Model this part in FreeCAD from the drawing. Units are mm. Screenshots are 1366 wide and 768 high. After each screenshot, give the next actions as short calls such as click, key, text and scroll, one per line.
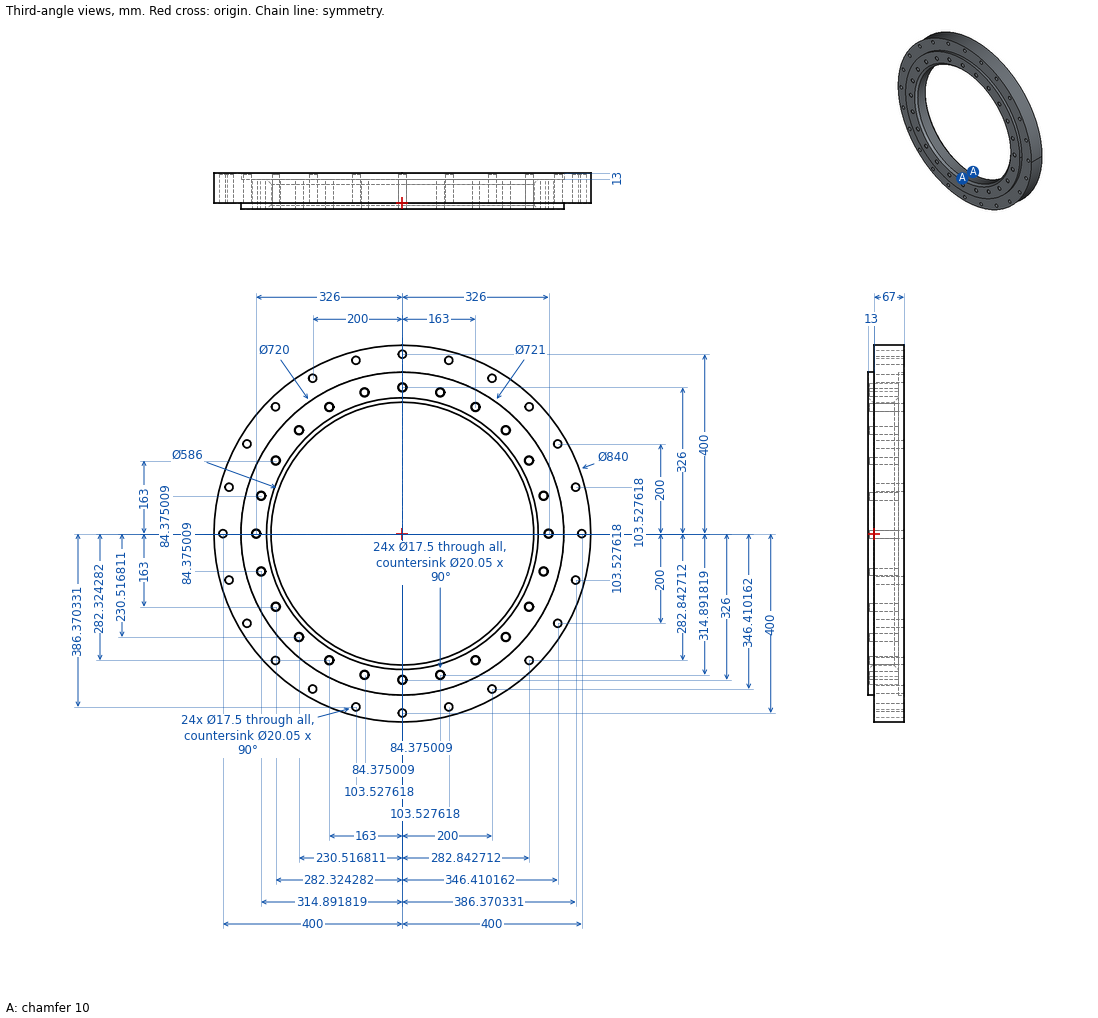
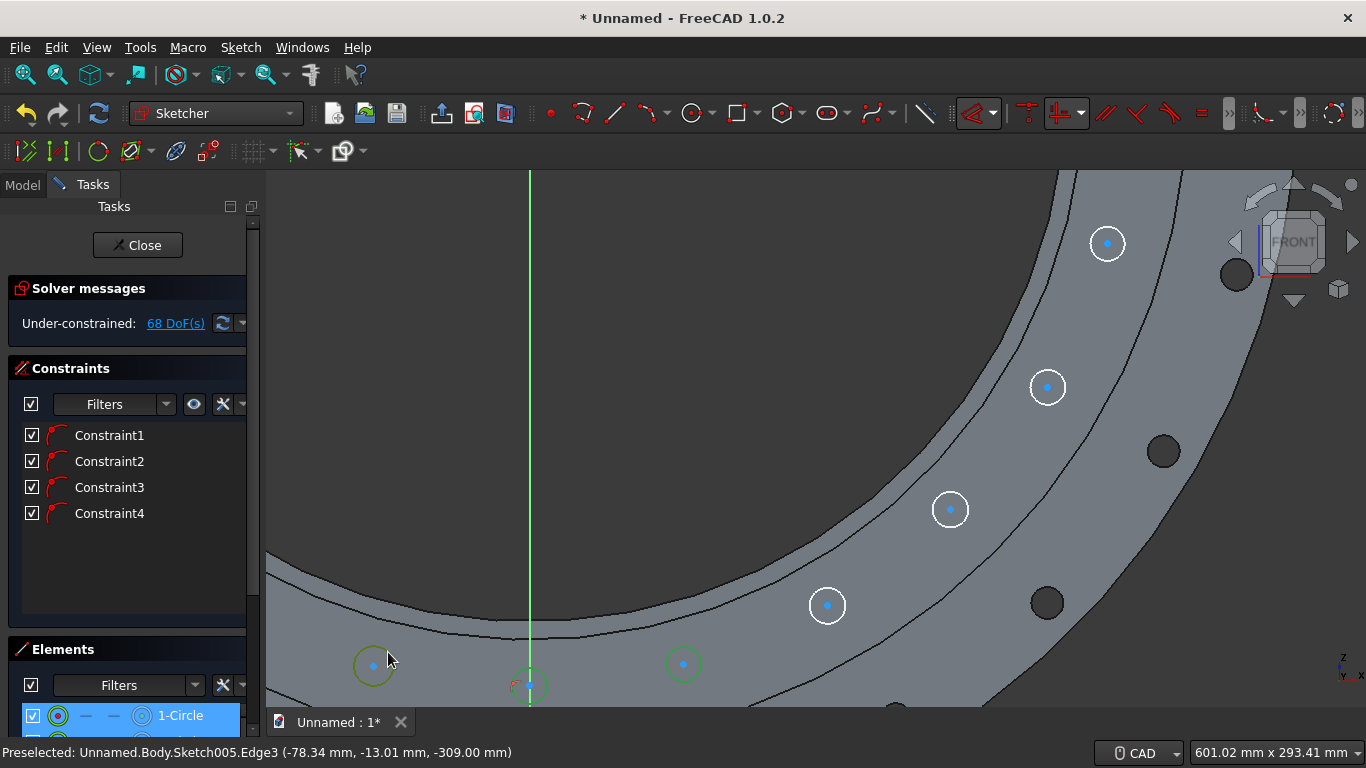
scroll(841, 591, down, 6)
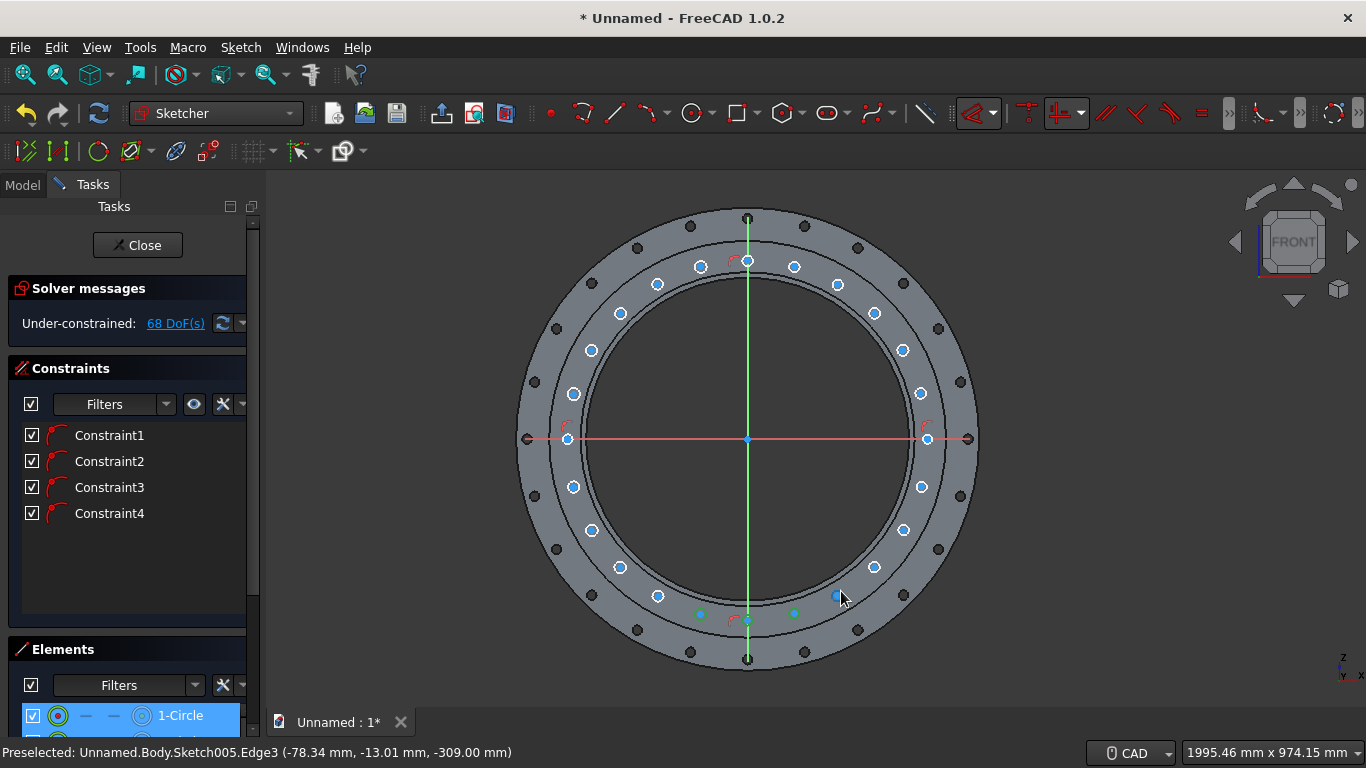
scroll(662, 592, up, 5)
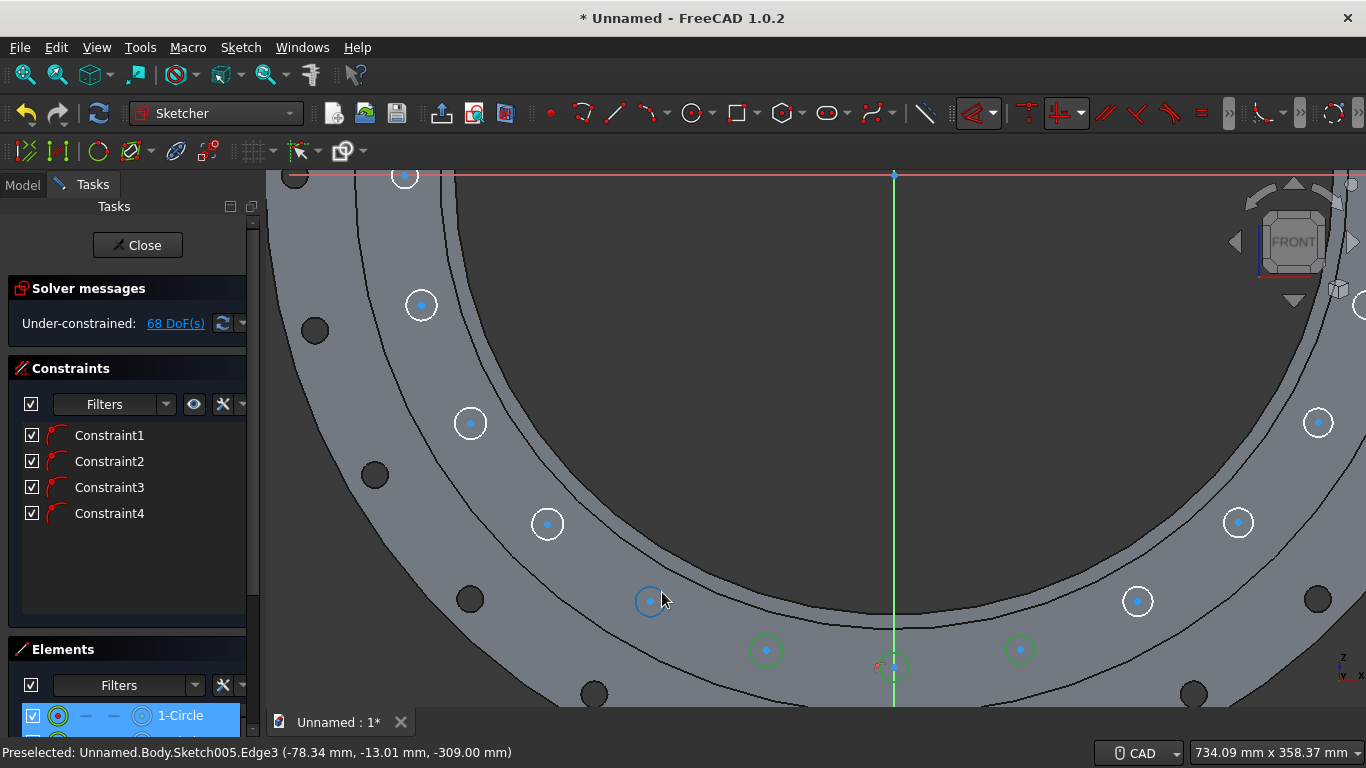
click(661, 591)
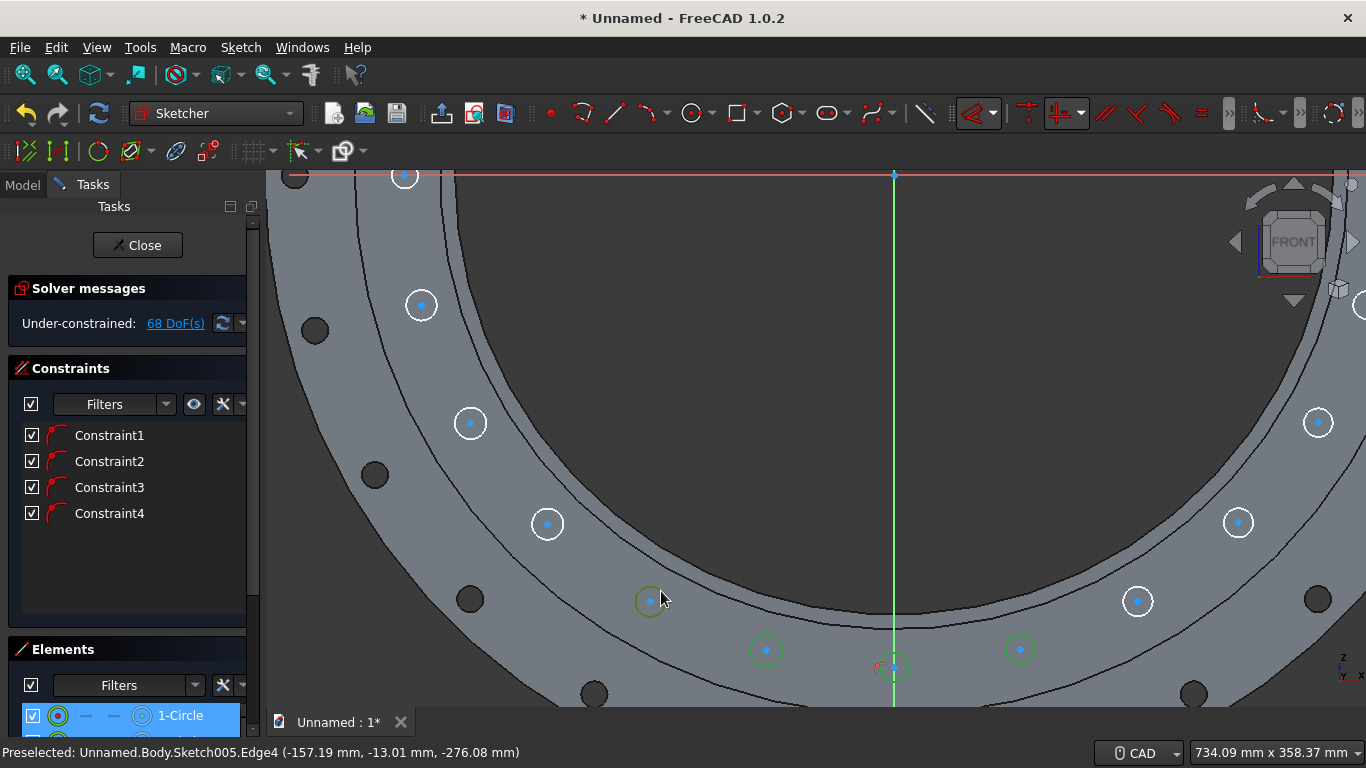
click(559, 513)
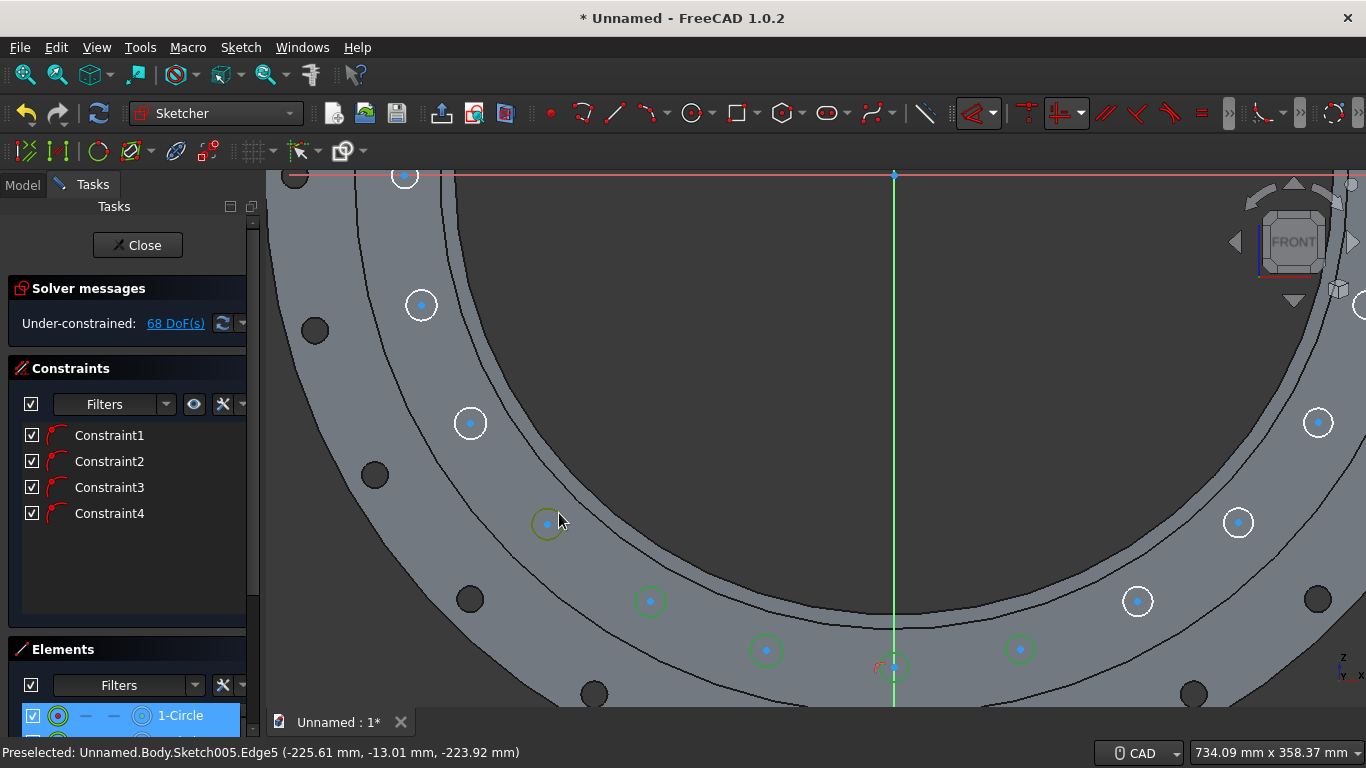
click(482, 412)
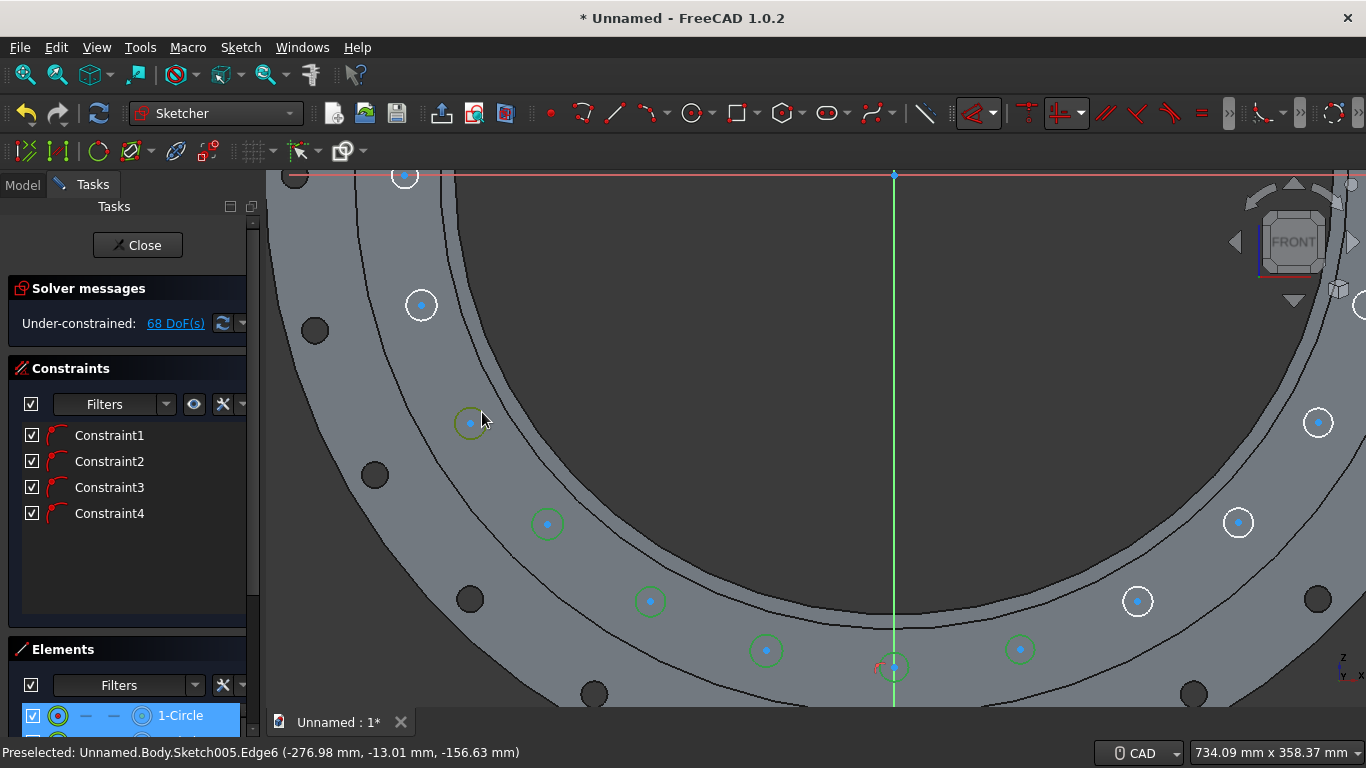
click(432, 295)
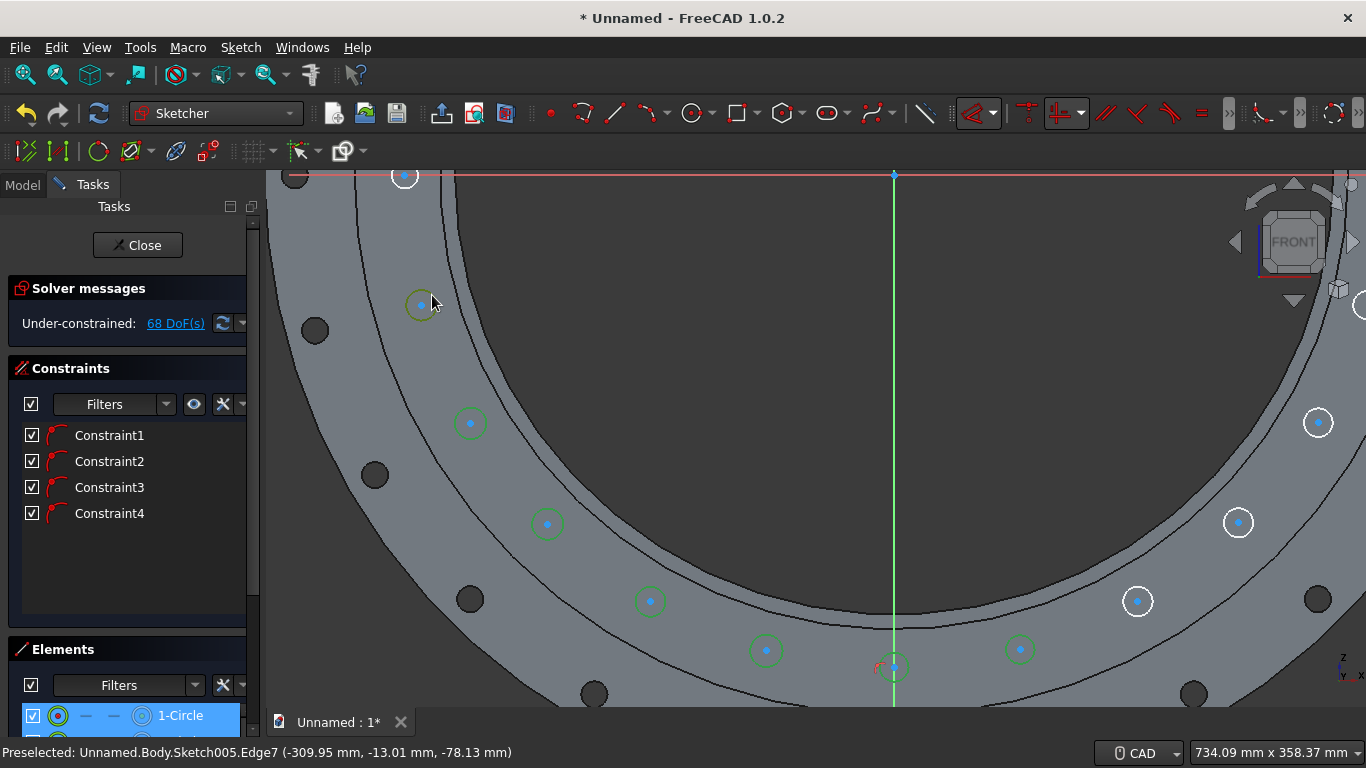
scroll(662, 592, down, 5)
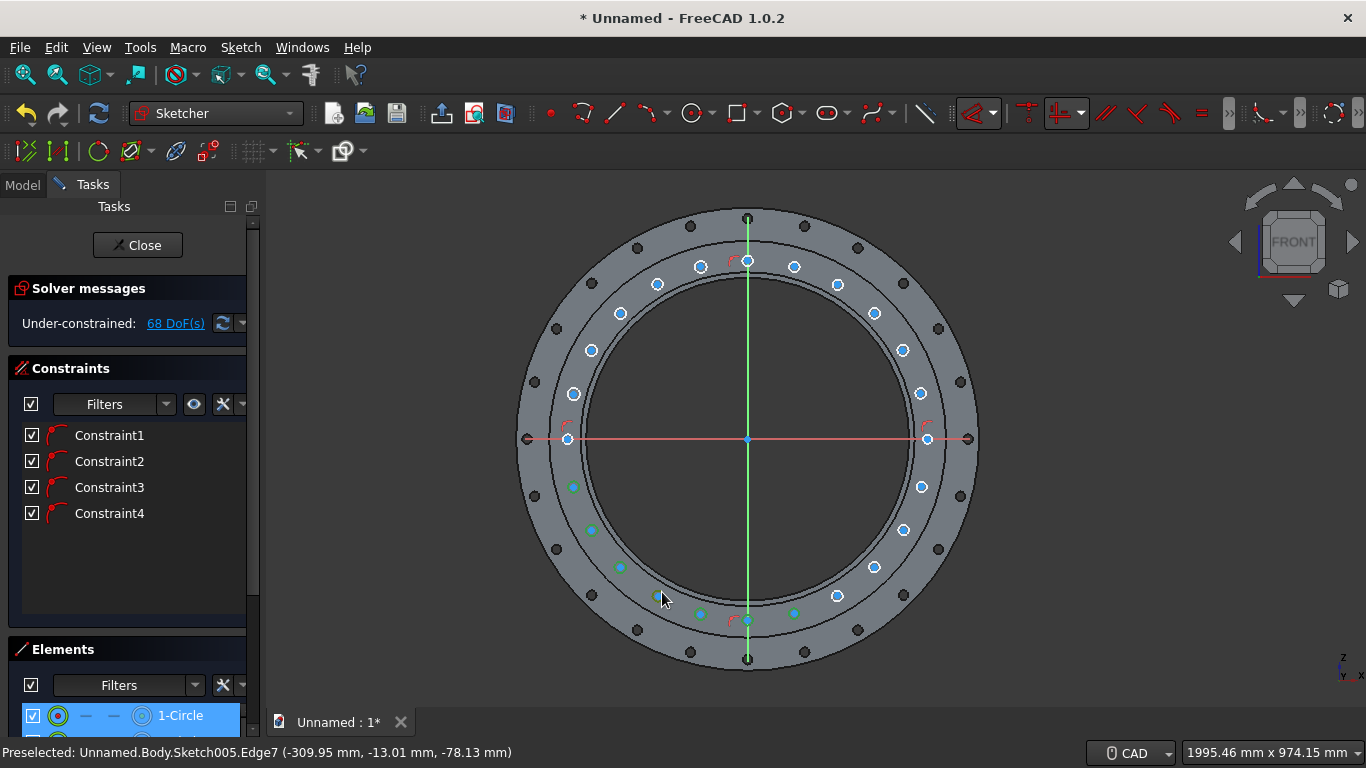
scroll(571, 436, up, 7)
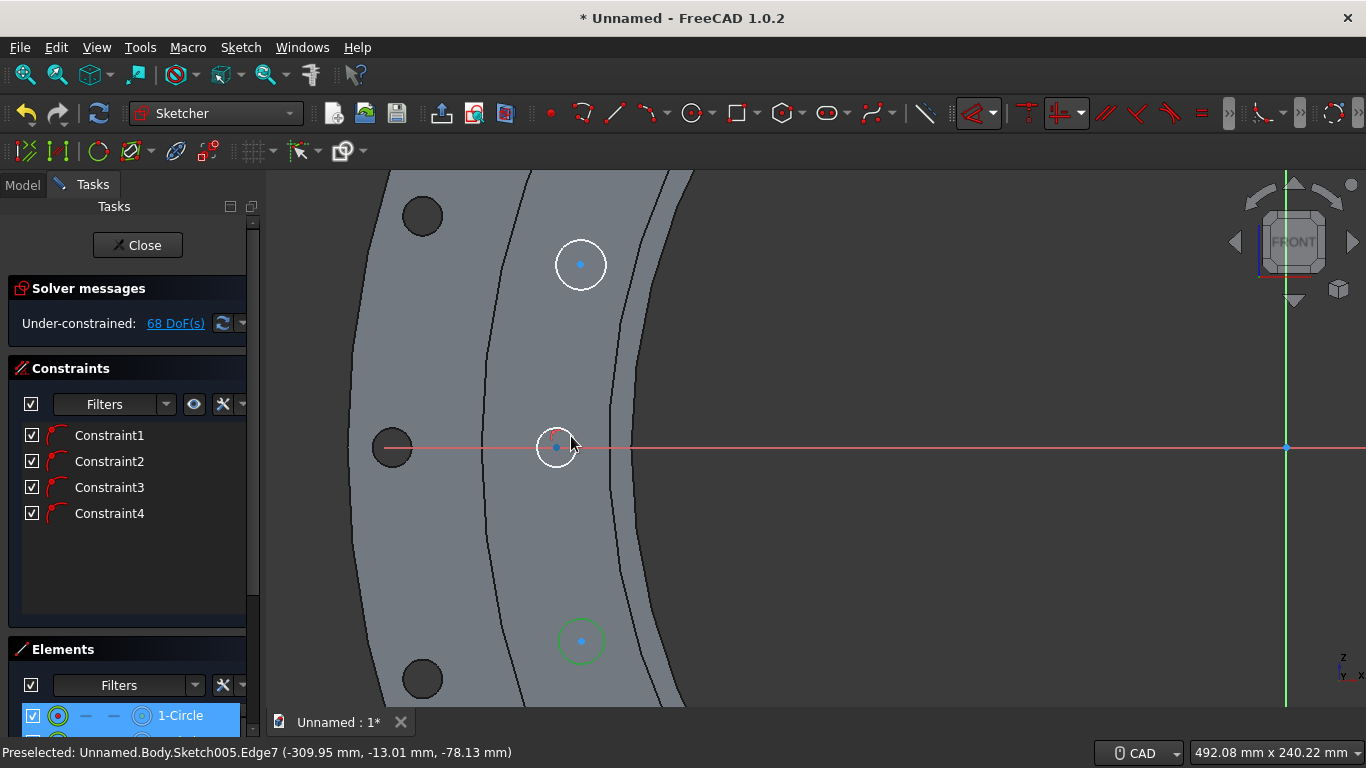
click(570, 434)